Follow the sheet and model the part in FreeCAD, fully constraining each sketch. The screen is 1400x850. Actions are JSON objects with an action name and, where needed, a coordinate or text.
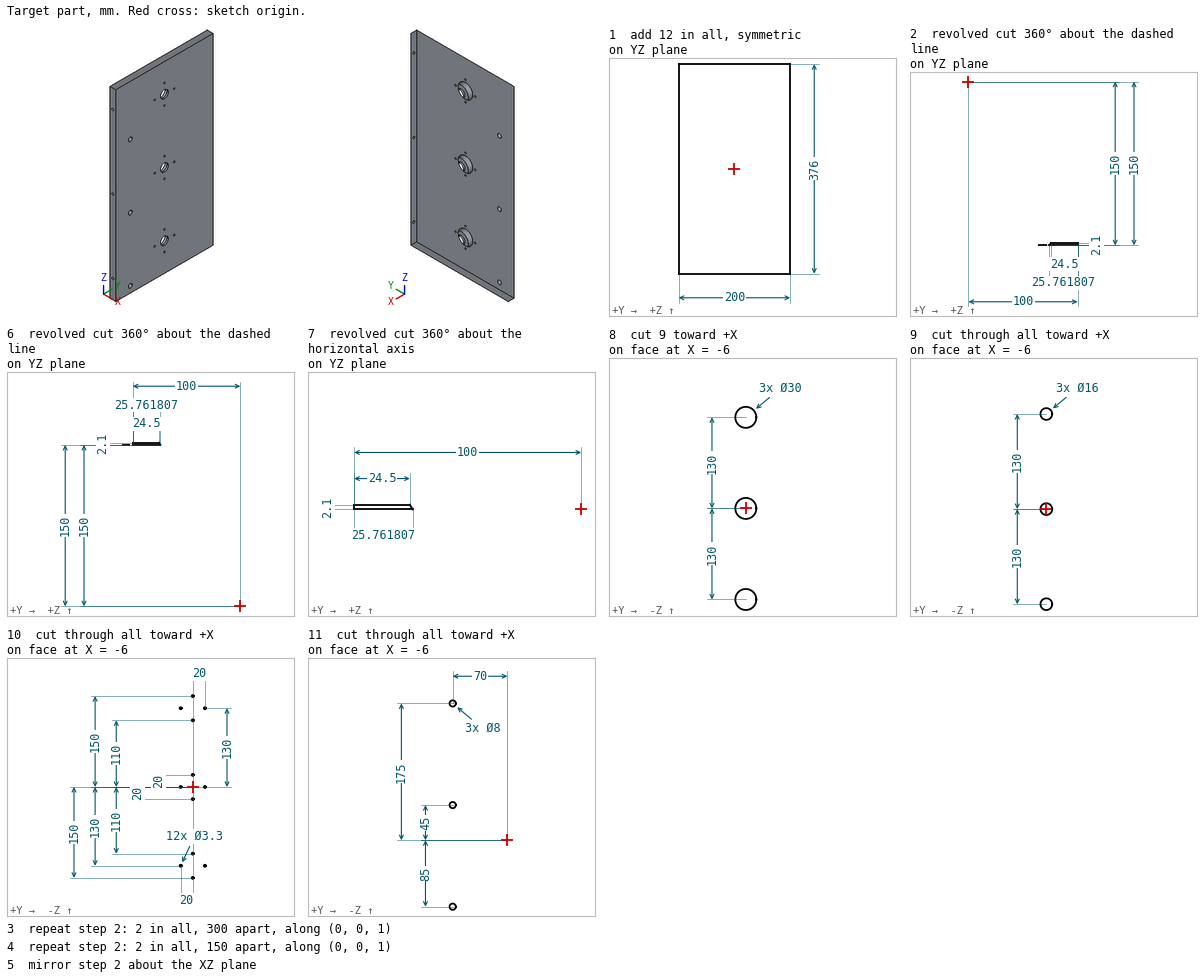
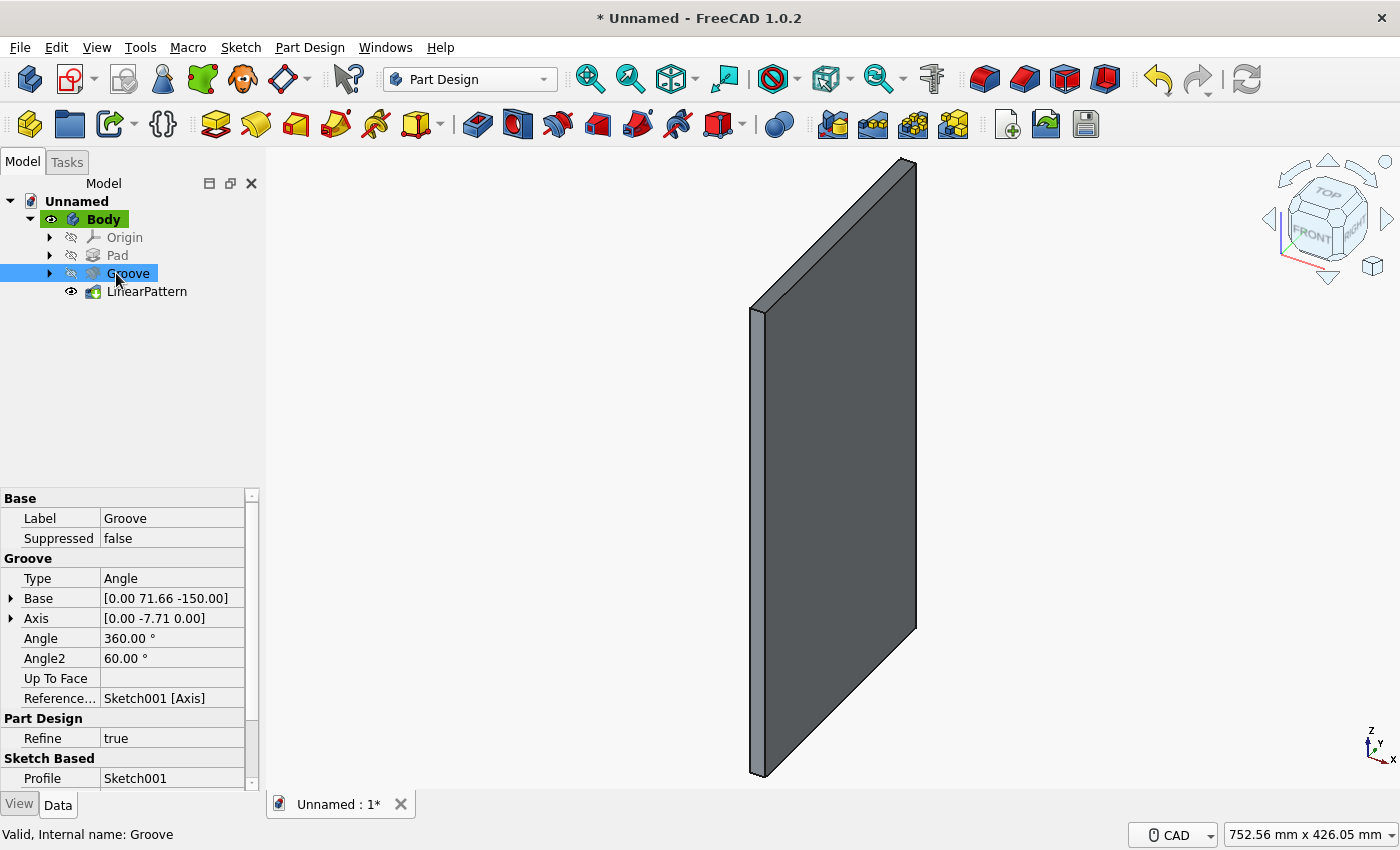
{"action": "left_click", "coordinate": [874, 124]}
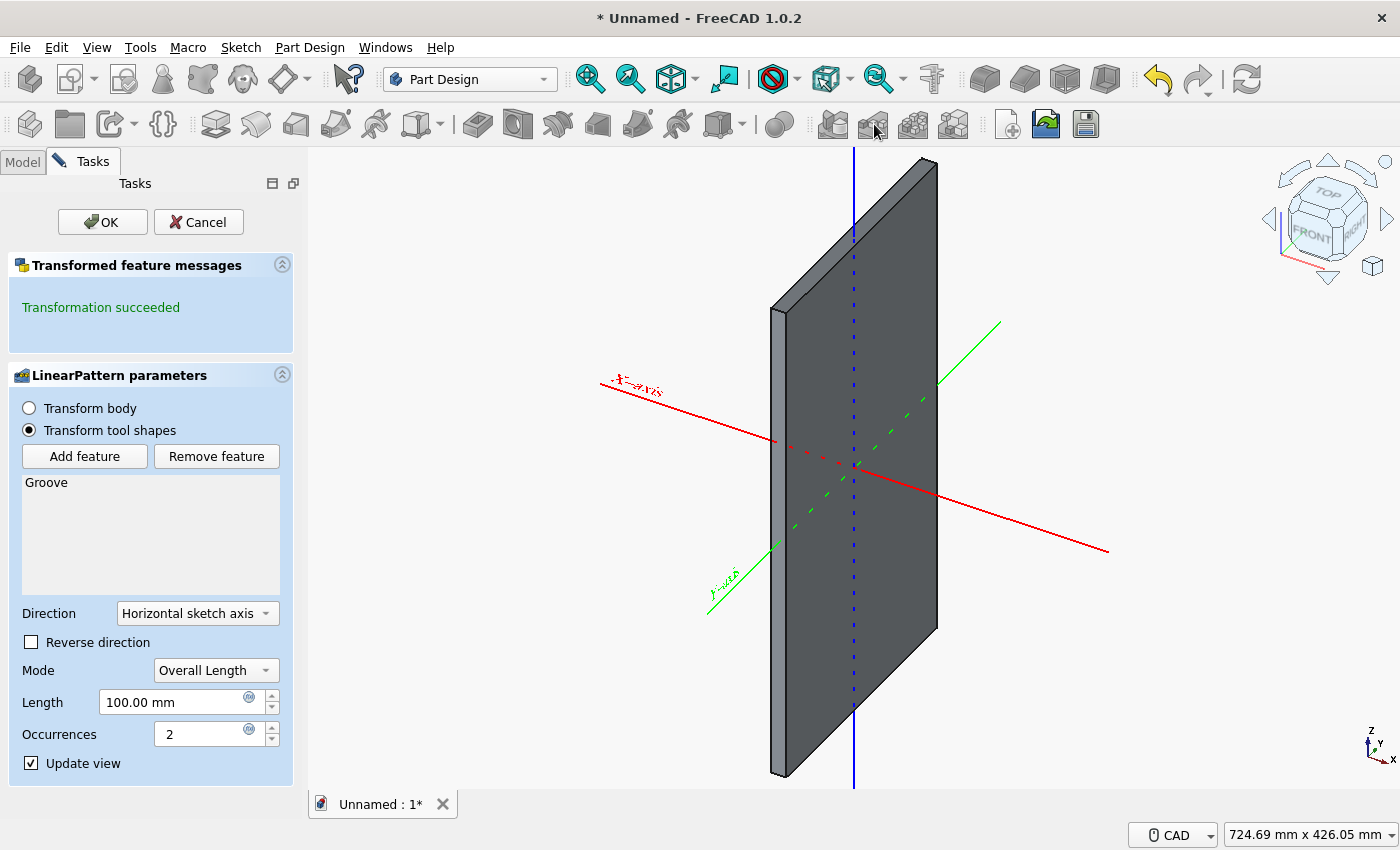
{"action": "left_click", "coordinate": [198, 614]}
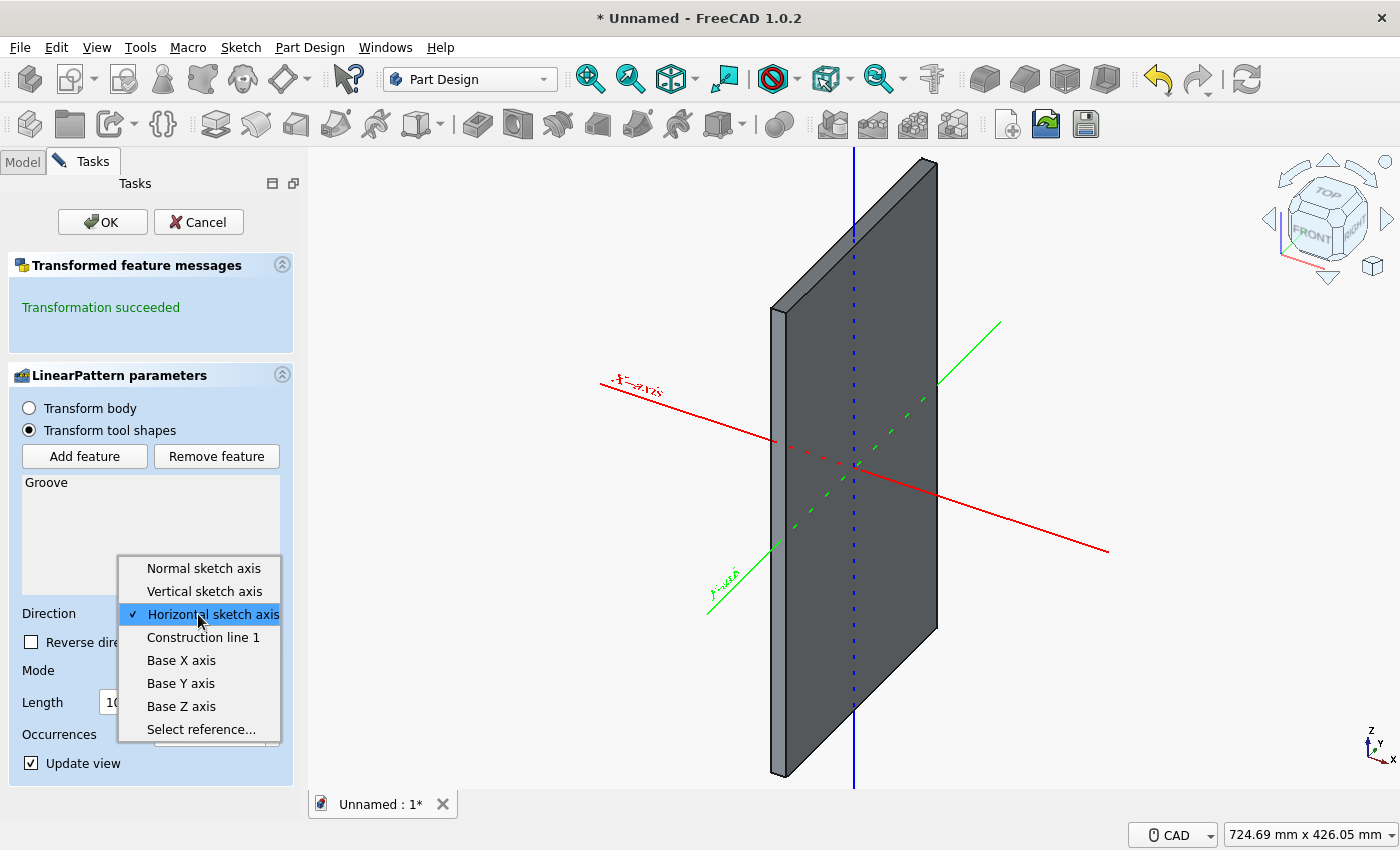
{"action": "left_click", "coordinate": [198, 706]}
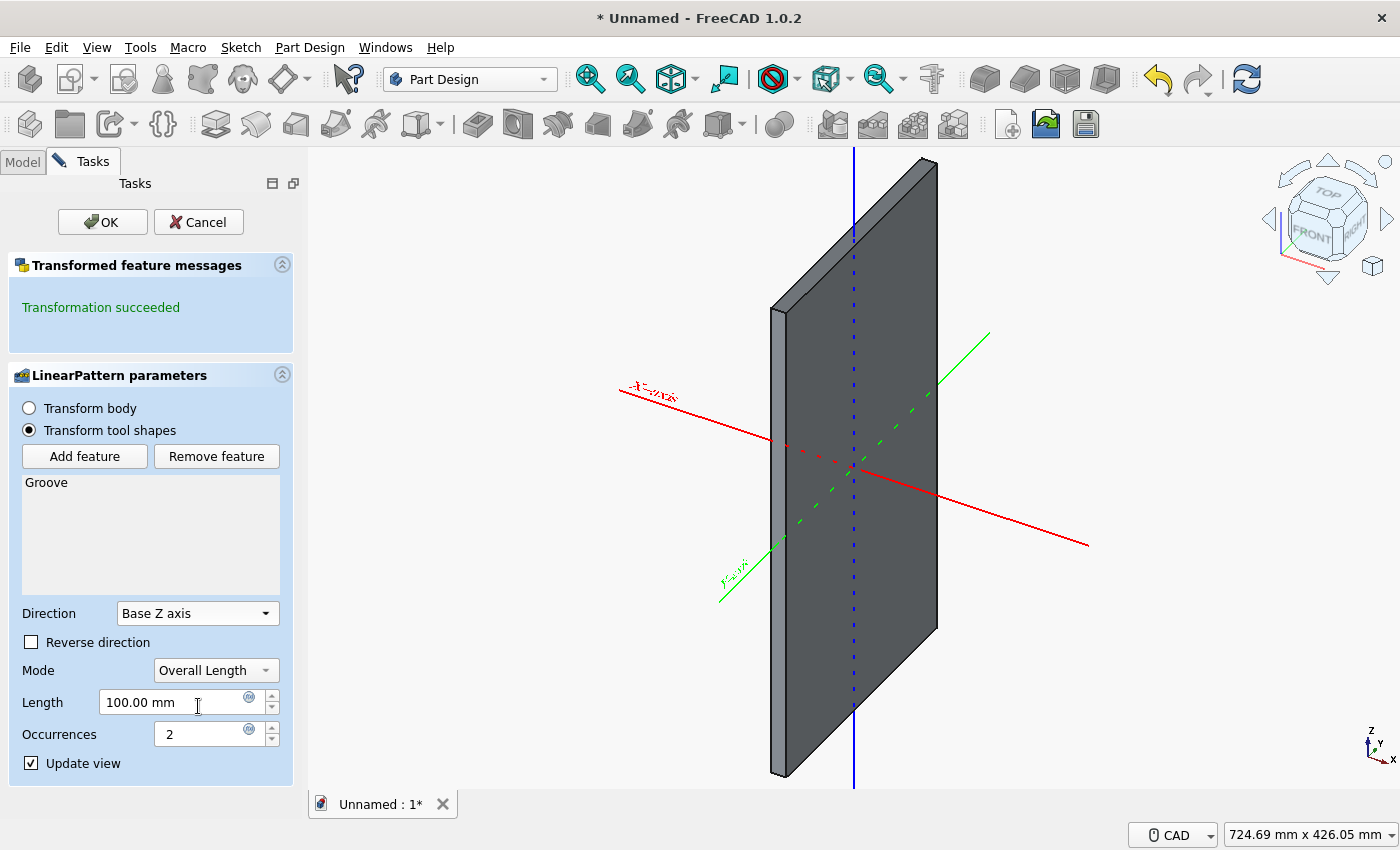
{"action": "left_click", "coordinate": [217, 670]}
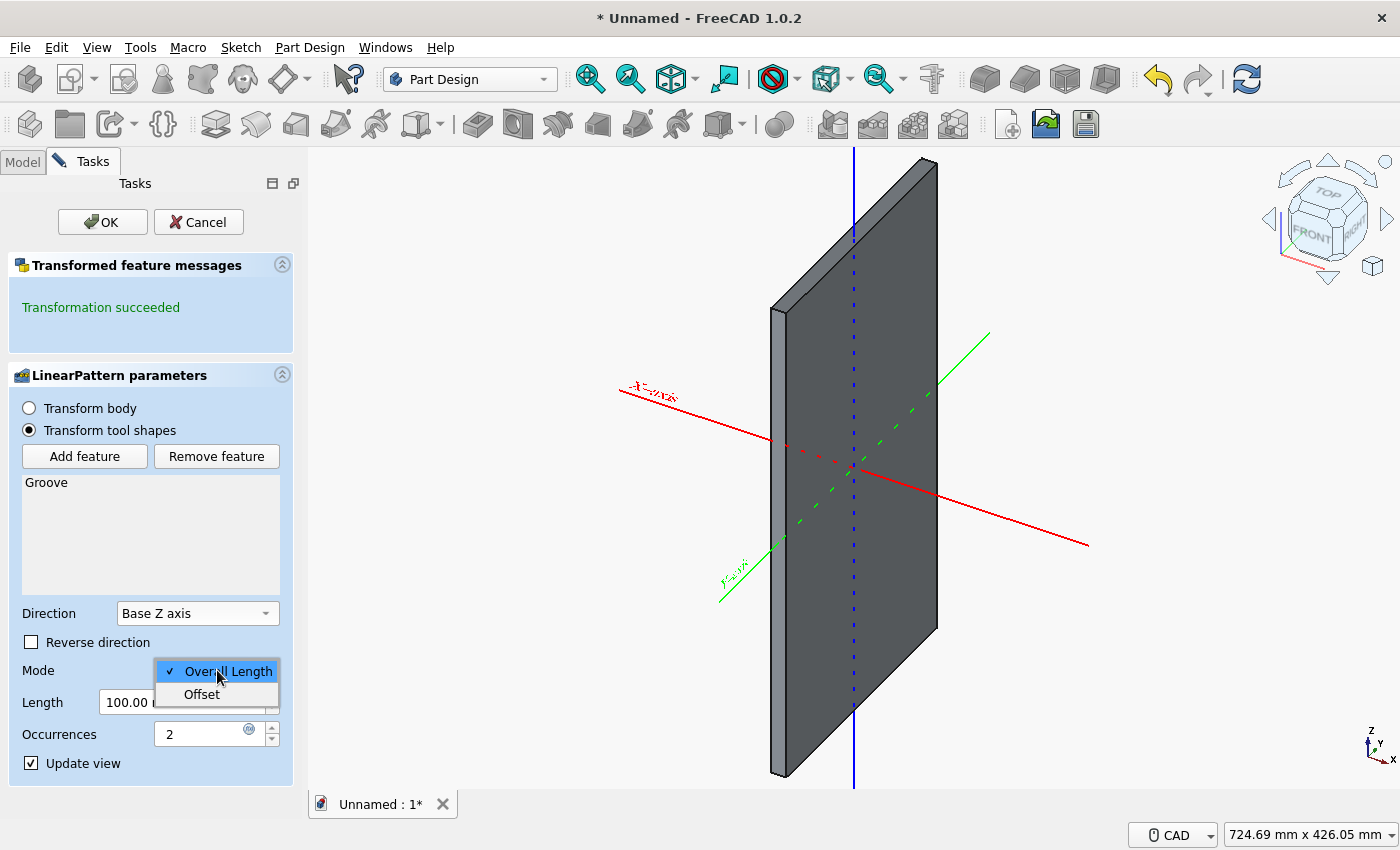
{"action": "left_click", "coordinate": [216, 694]}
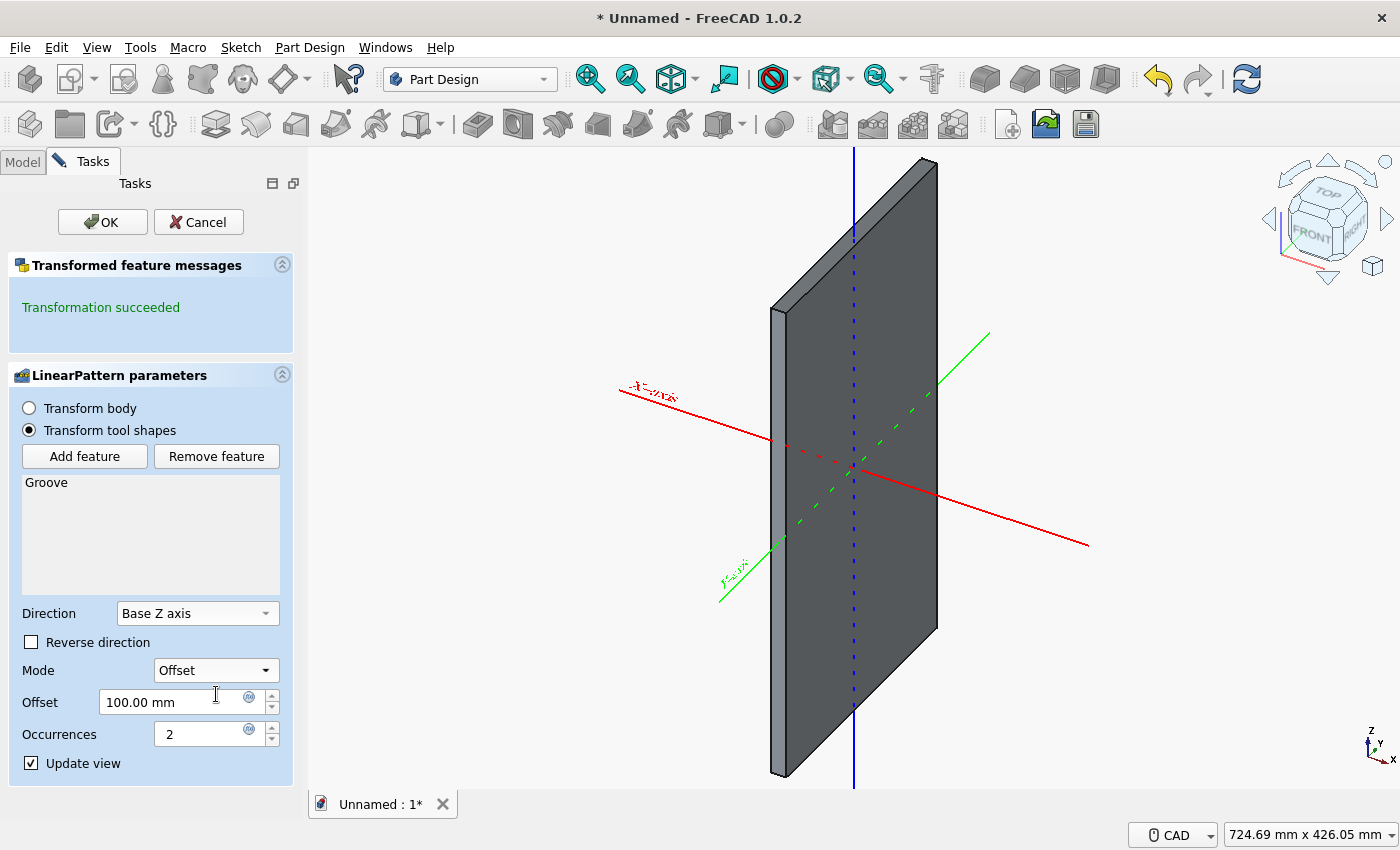
{"action": "triple_click", "coordinate": [182, 702]}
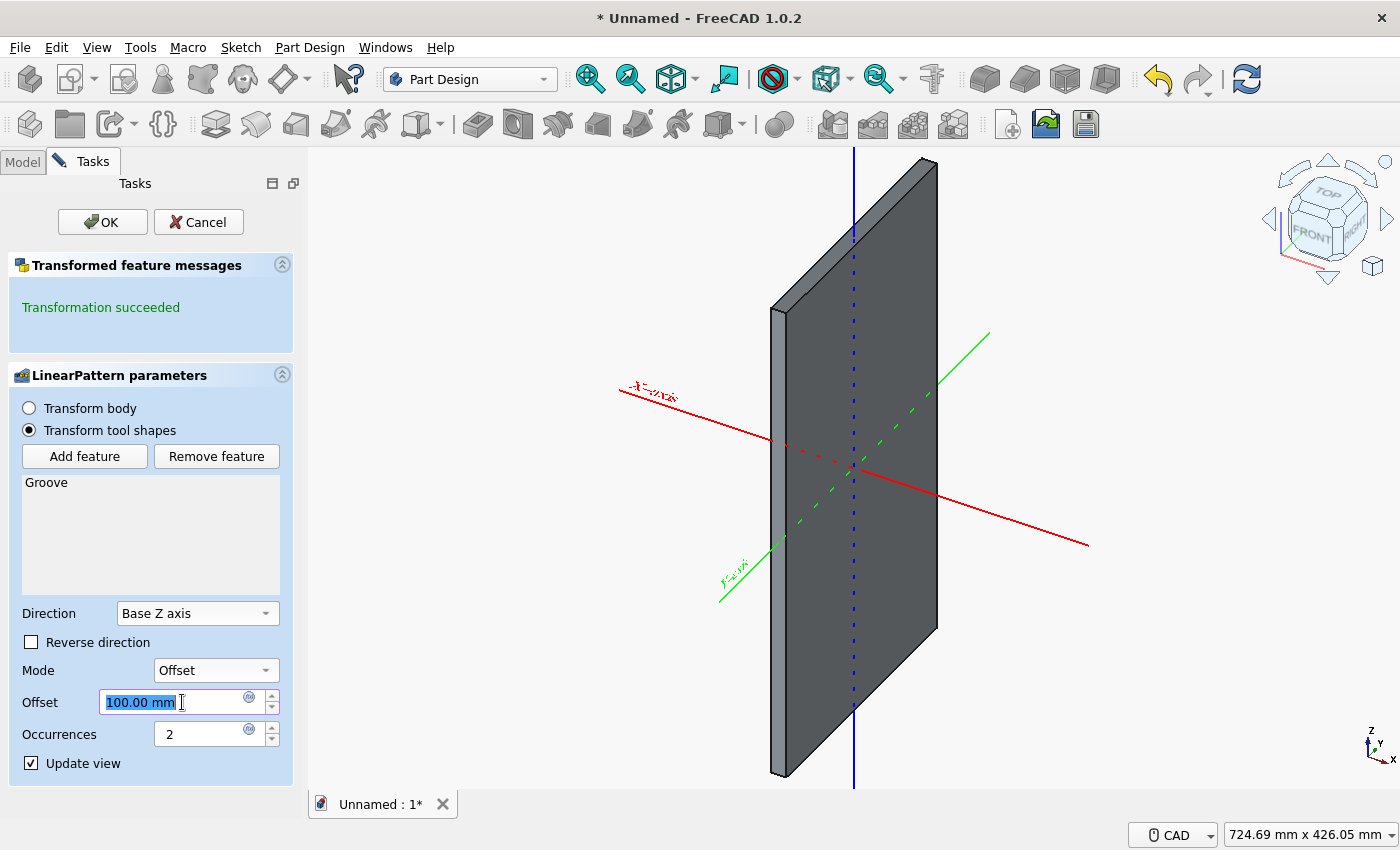
{"action": "type", "text": "150"}
{"action": "key", "text": "Tab"}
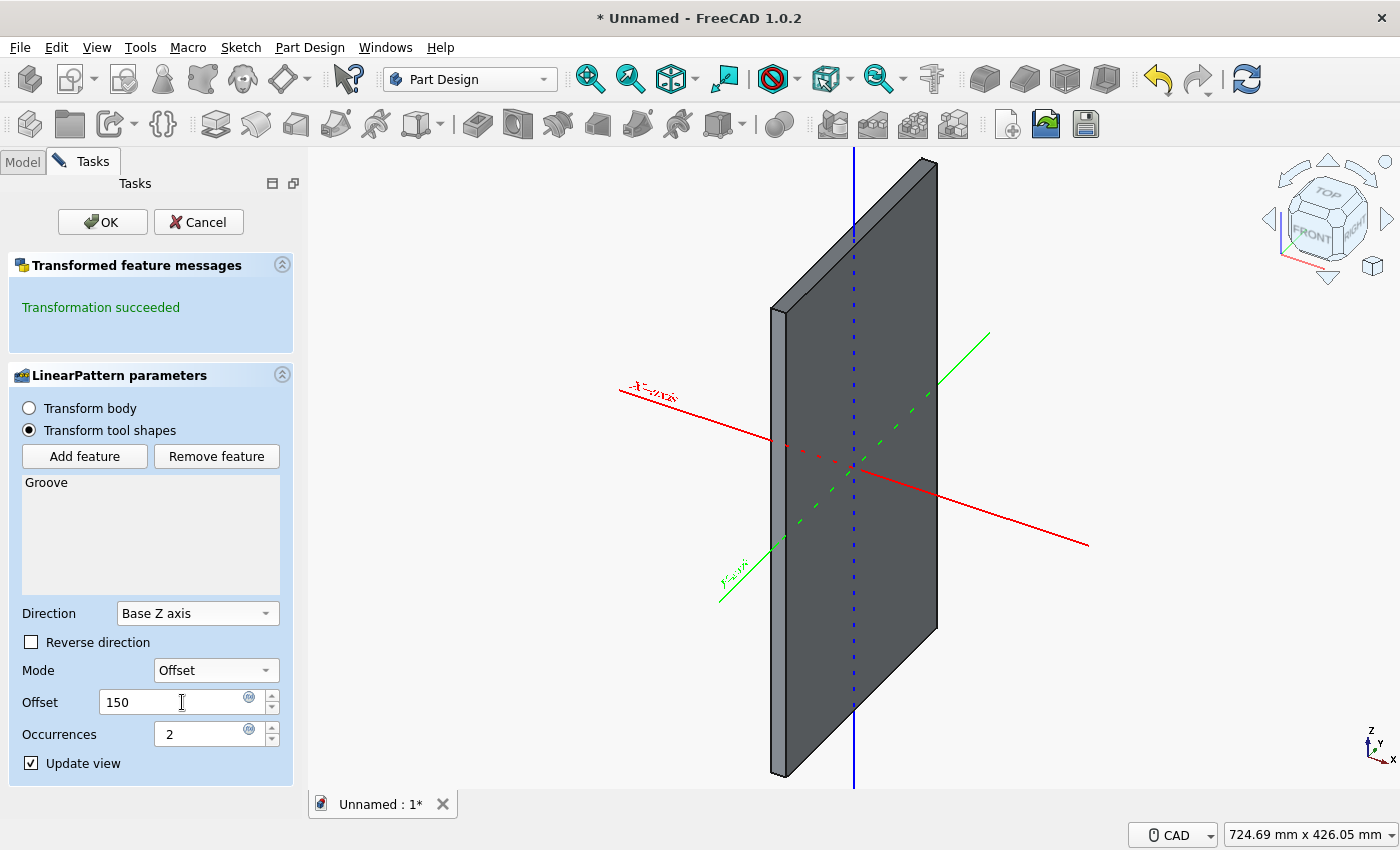
{"action": "triple_click", "coordinate": [209, 734]}